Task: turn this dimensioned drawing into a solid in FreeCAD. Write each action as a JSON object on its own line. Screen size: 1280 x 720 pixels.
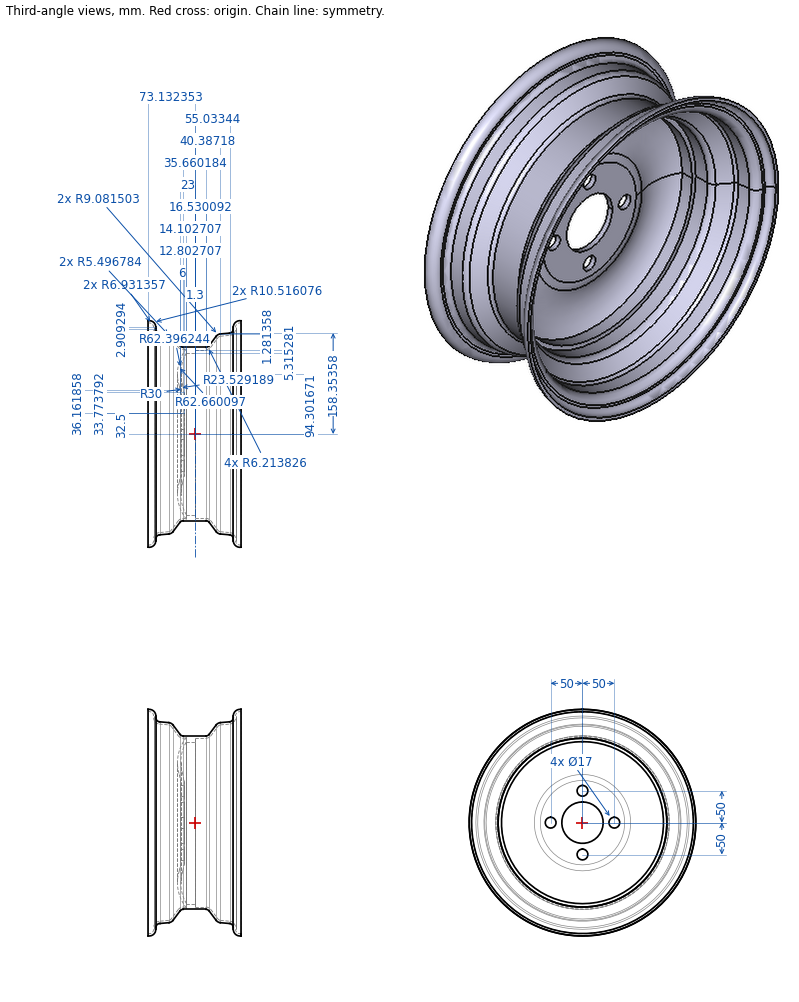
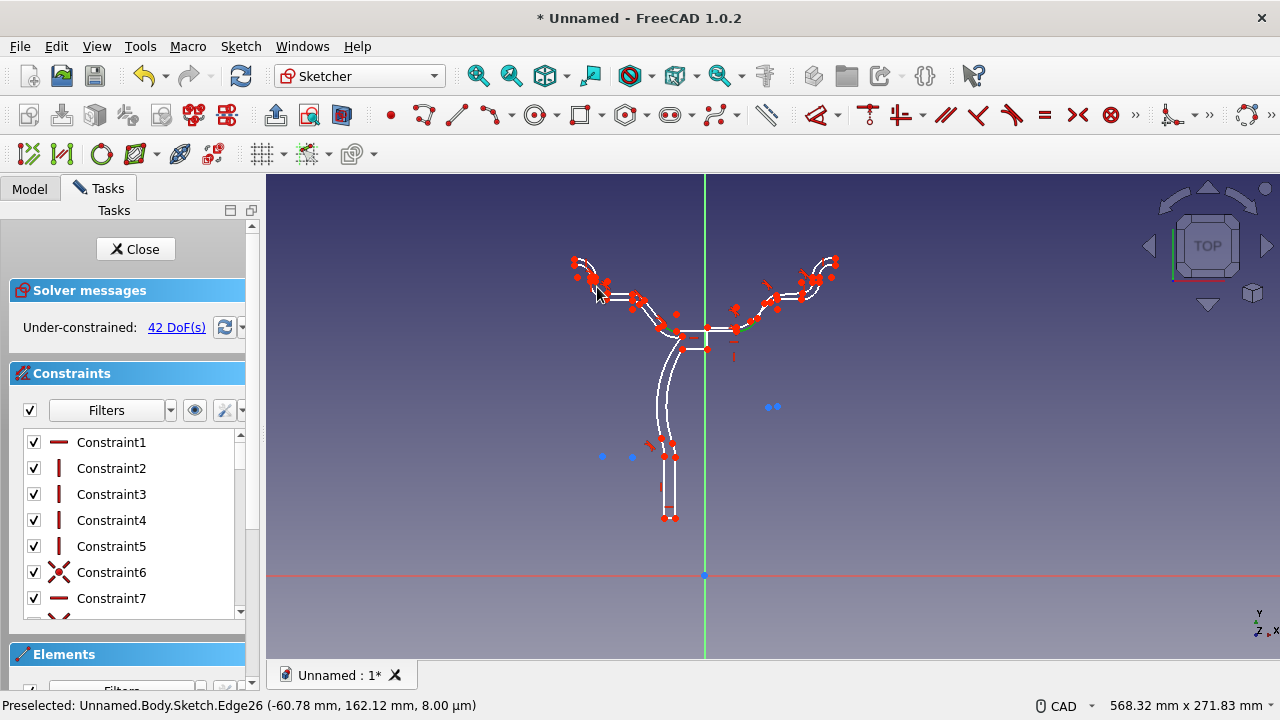
{"action": "scroll", "coordinate": [807, 292], "scroll_direction": "up", "scroll_amount": 6}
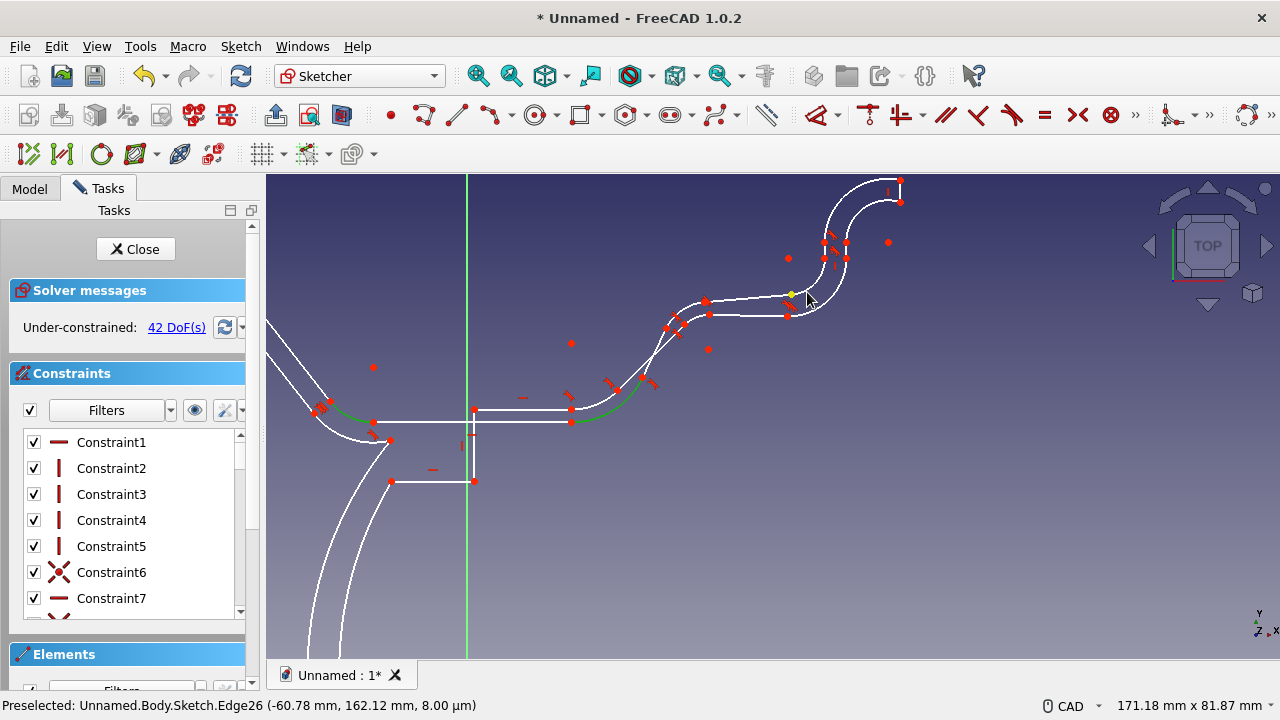
{"action": "left_click", "coordinate": [807, 290]}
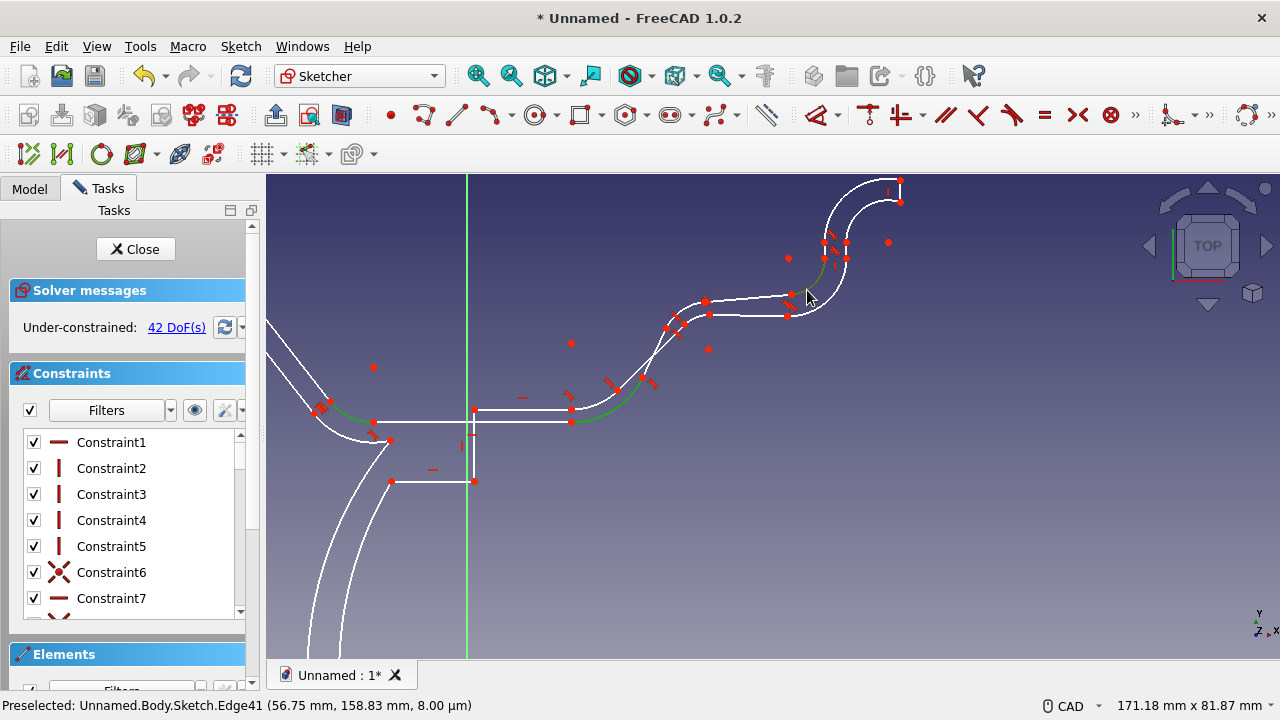
{"action": "key", "text": "e"}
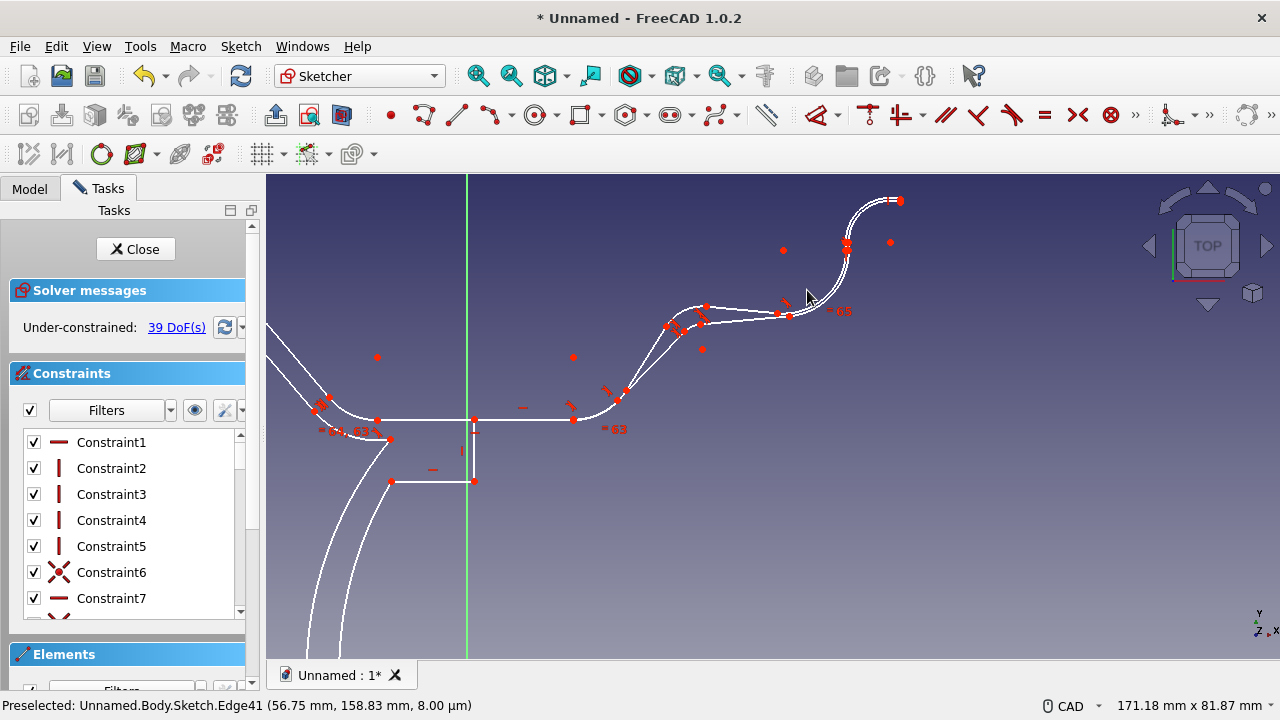
{"action": "left_click", "coordinate": [692, 308]}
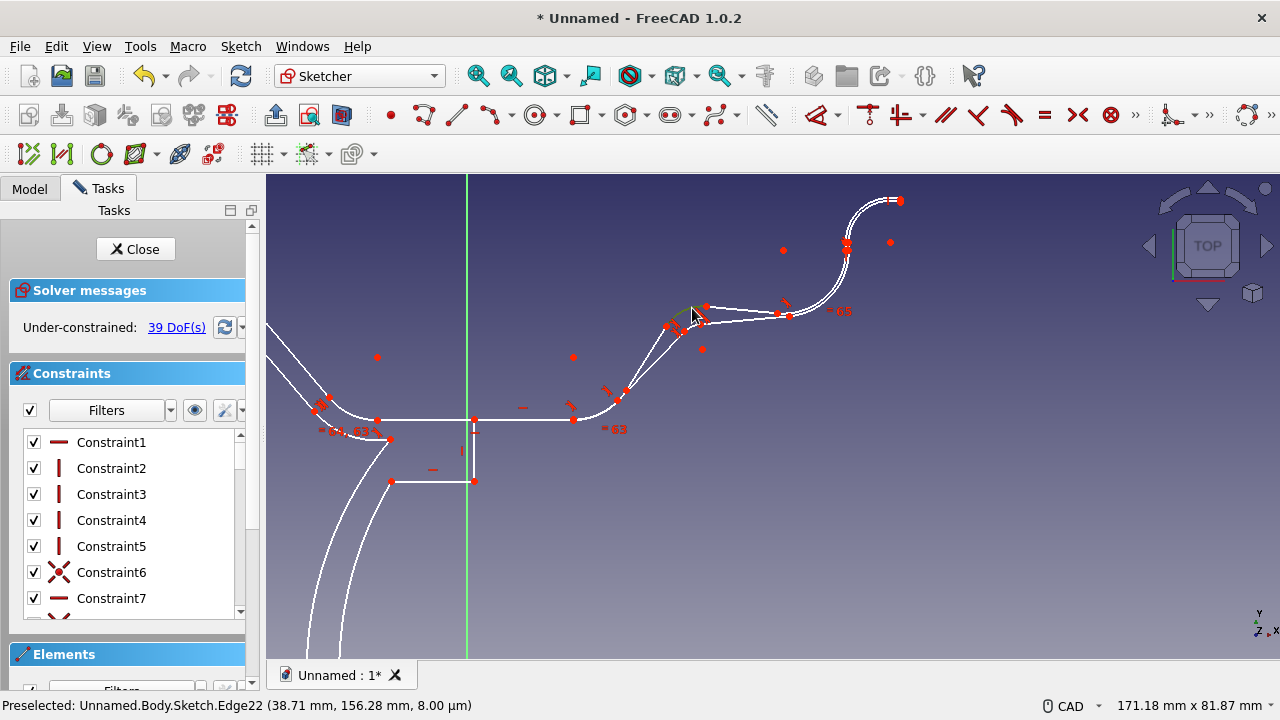
{"action": "scroll", "coordinate": [807, 292], "scroll_direction": "down", "scroll_amount": 6}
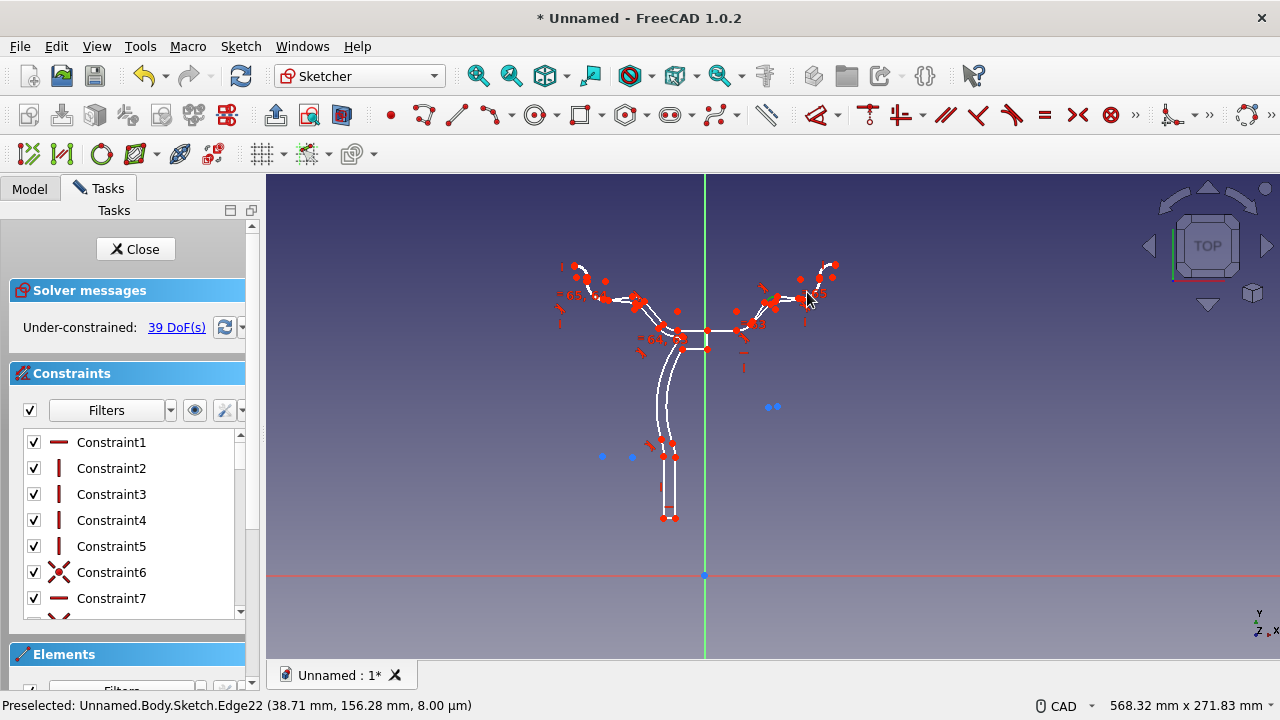
{"action": "scroll", "coordinate": [641, 299], "scroll_direction": "up", "scroll_amount": 7}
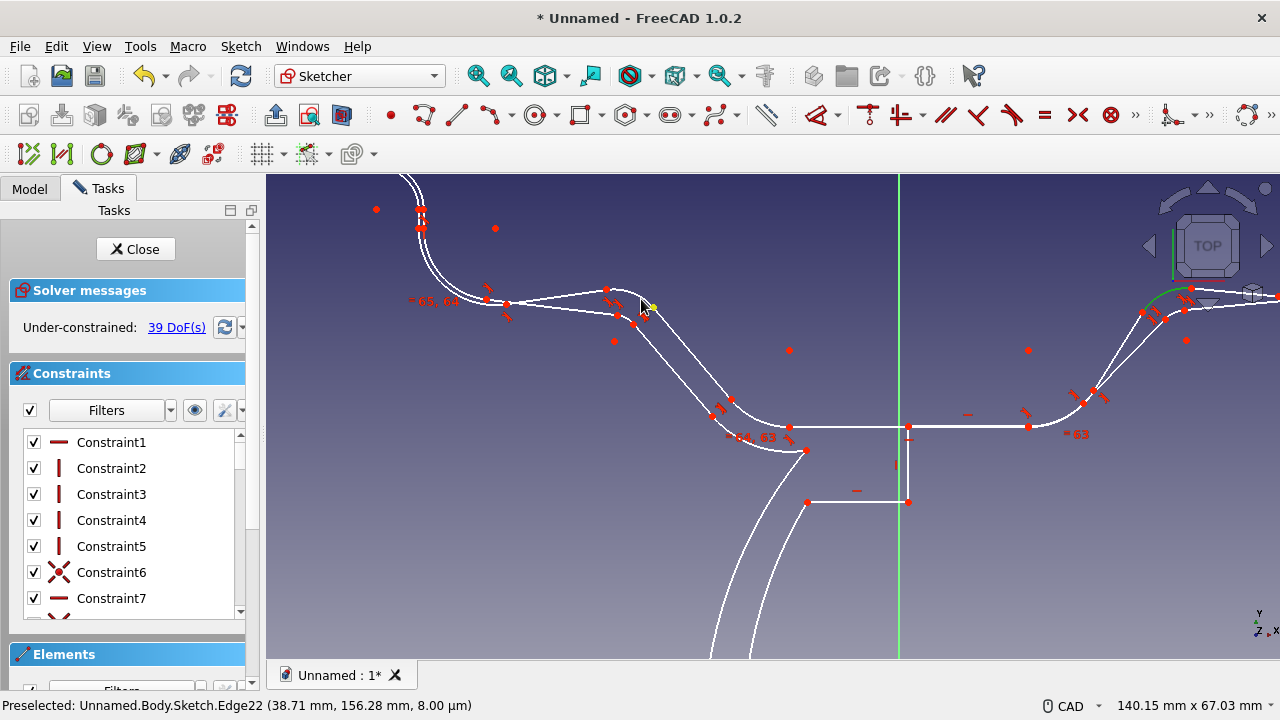
{"action": "left_click", "coordinate": [642, 298]}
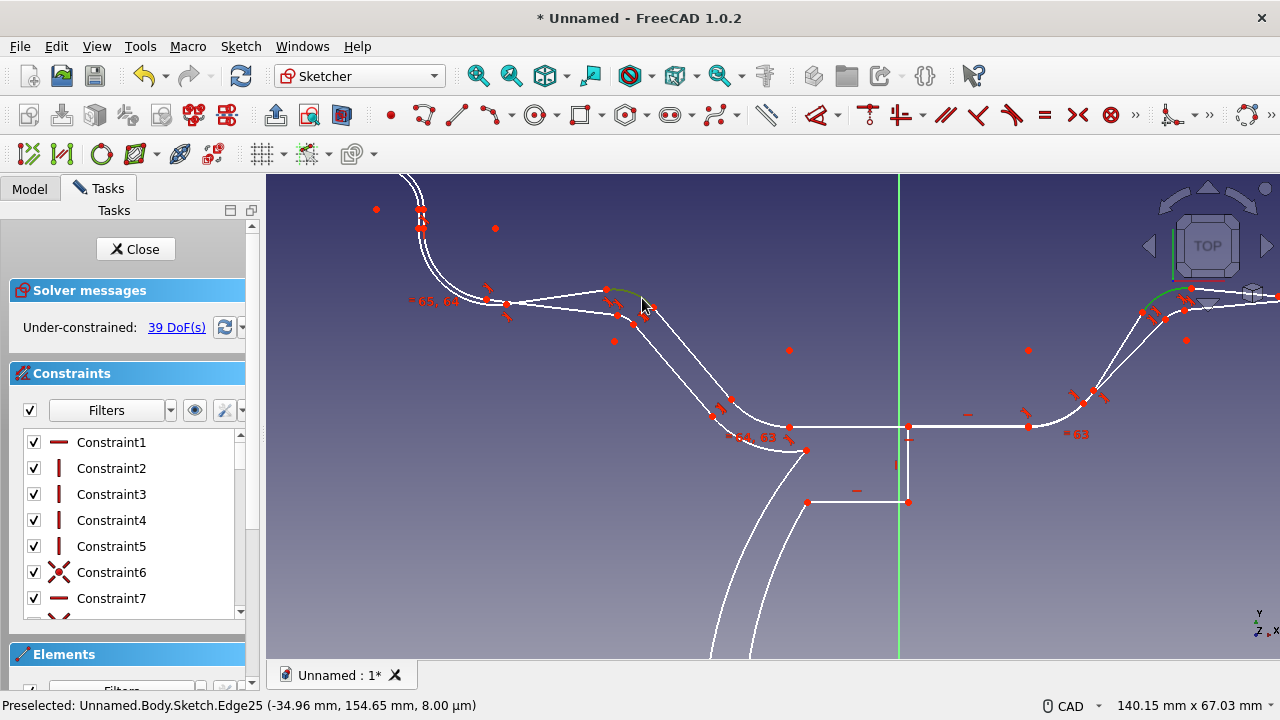
{"action": "left_click", "coordinate": [1045, 116]}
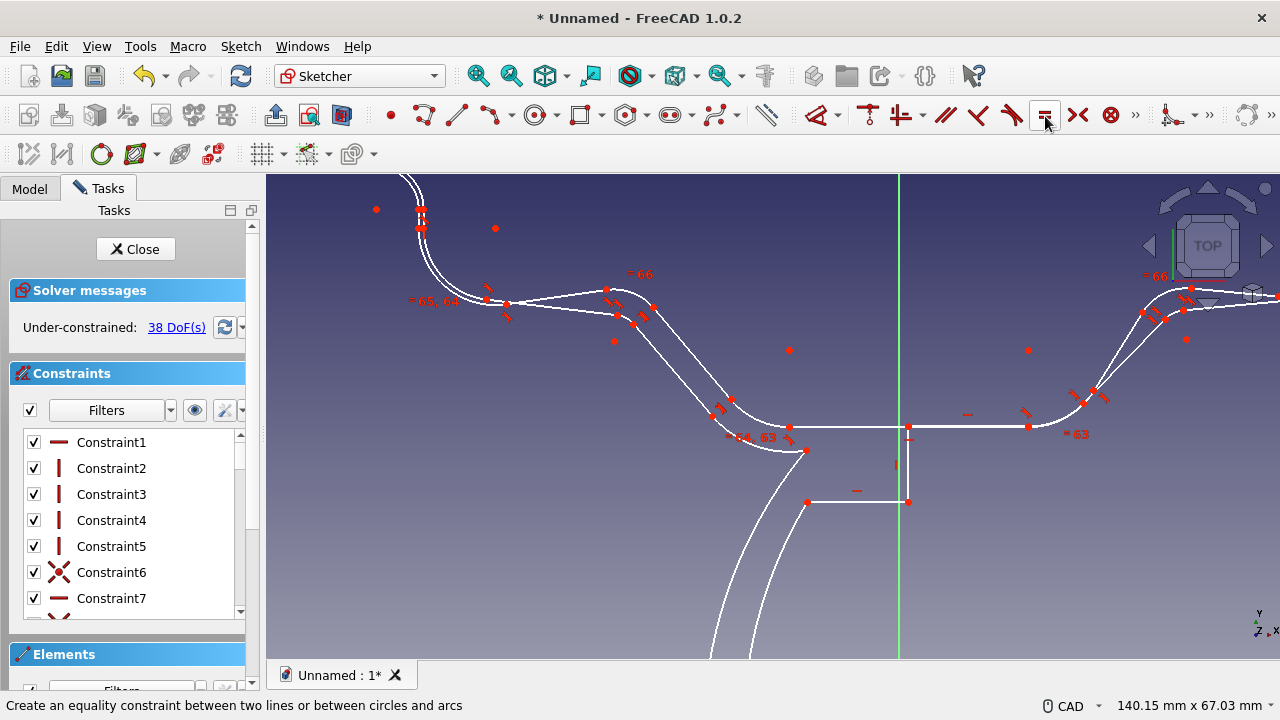
{"action": "scroll", "coordinate": [430, 259], "scroll_direction": "up", "scroll_amount": 6}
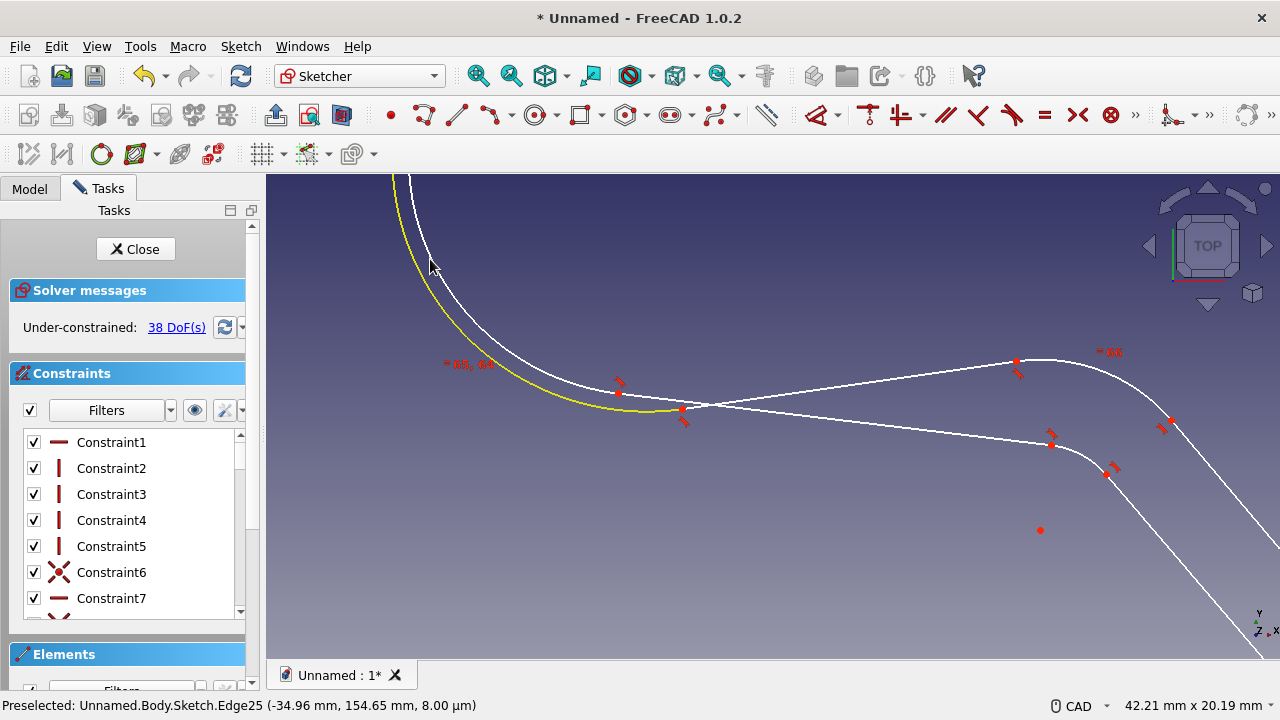
{"action": "left_click", "coordinate": [431, 258]}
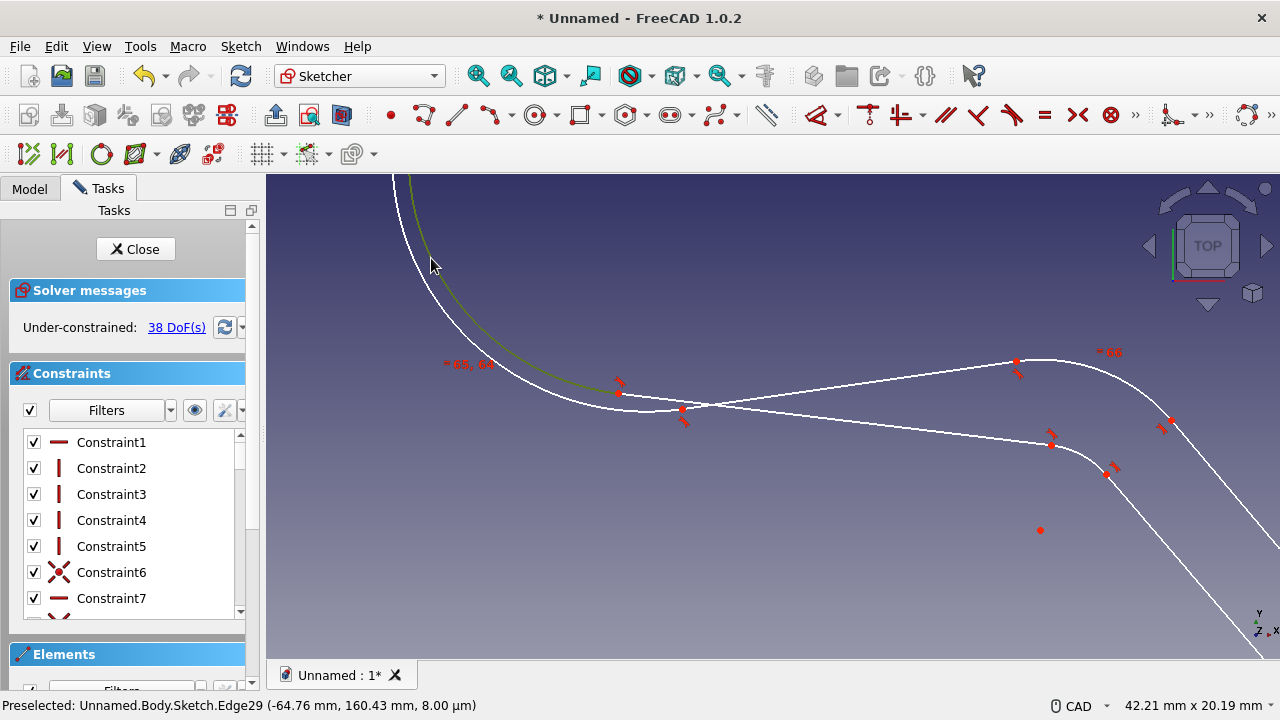
{"action": "scroll", "coordinate": [602, 291], "scroll_direction": "down", "scroll_amount": 13}